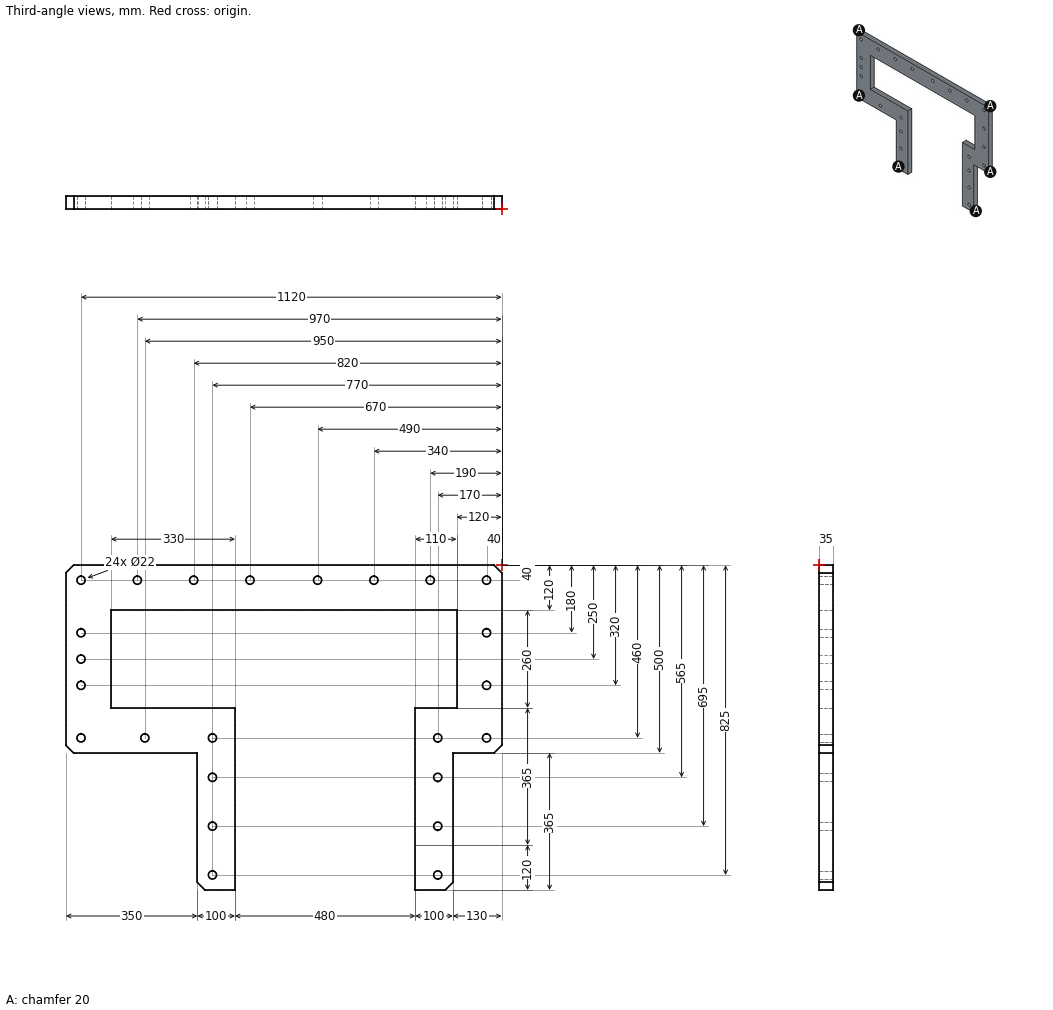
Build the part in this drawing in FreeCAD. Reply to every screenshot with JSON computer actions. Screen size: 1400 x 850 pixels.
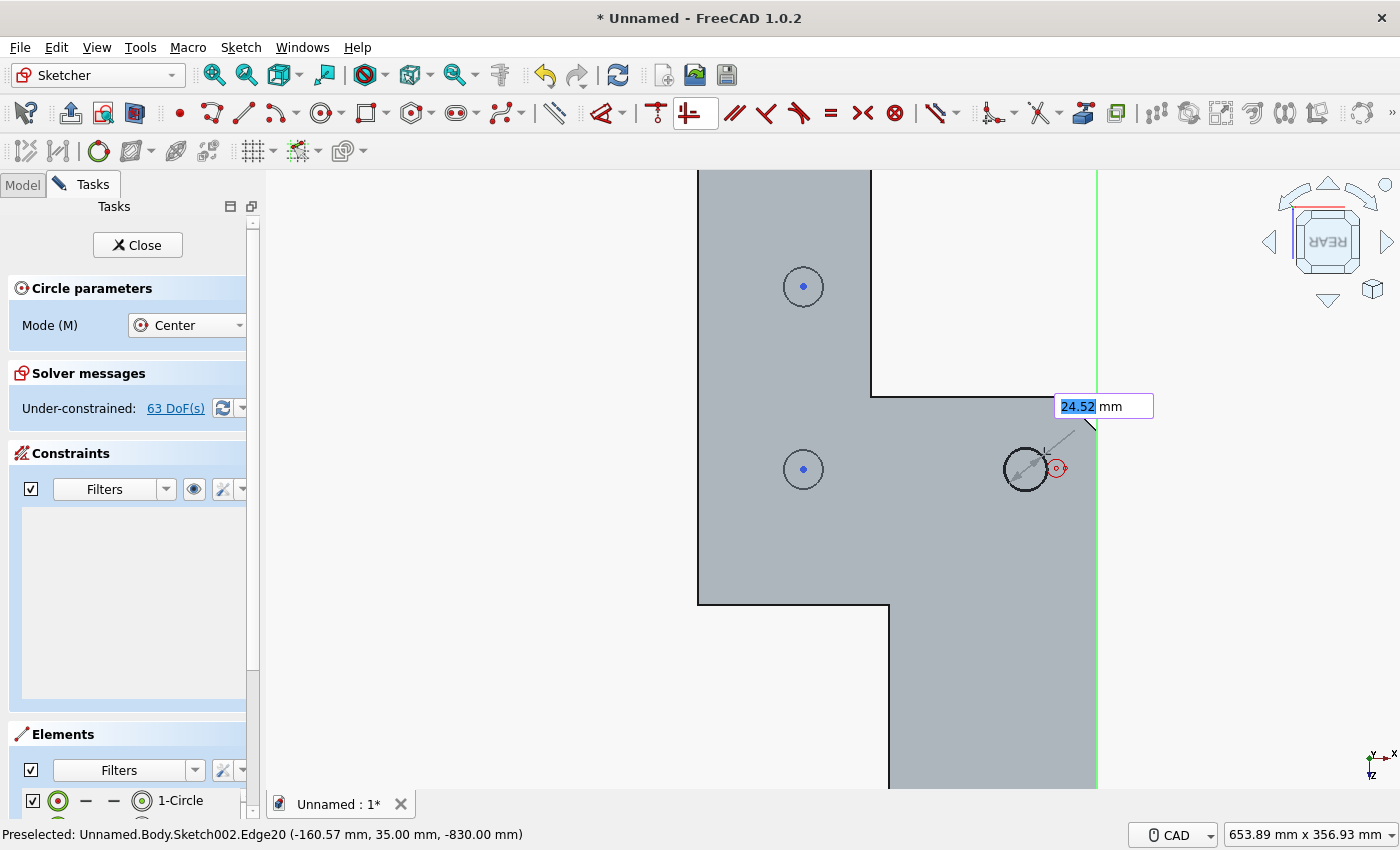
{"action": "left_click", "coordinate": [1041, 453]}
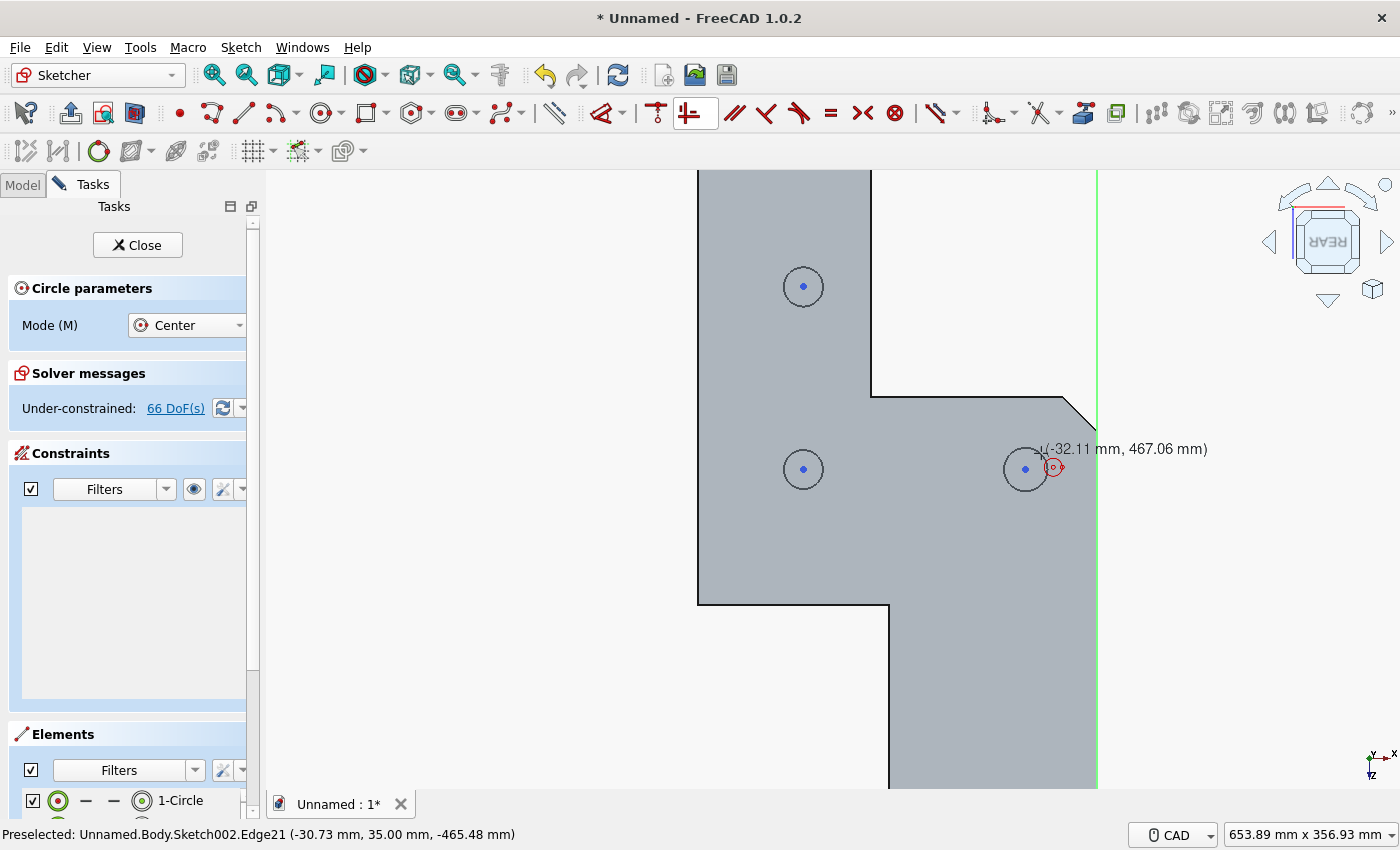
{"action": "scroll", "coordinate": [1044, 454], "scroll_direction": "down", "scroll_amount": 6}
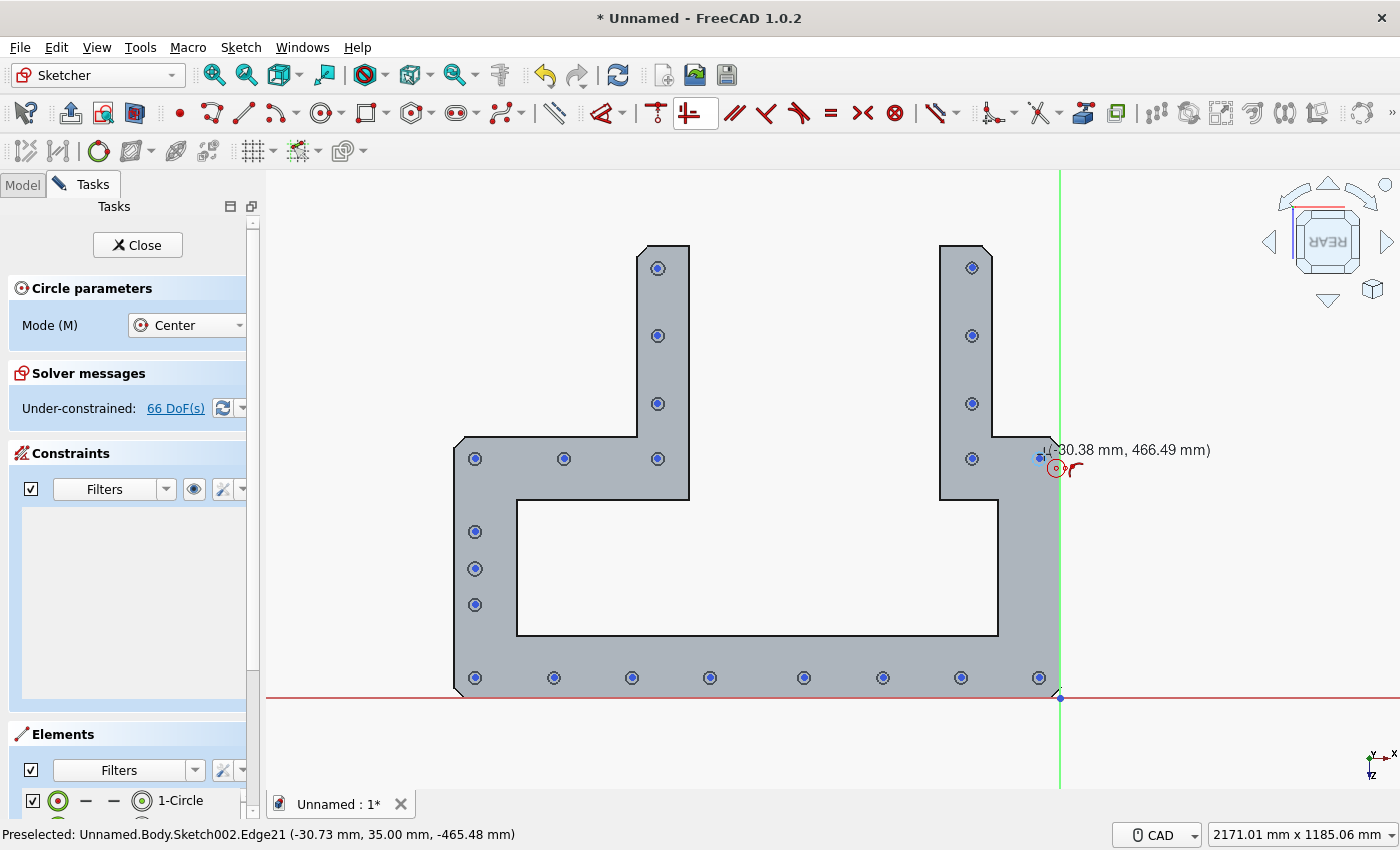
{"action": "left_click", "coordinate": [1039, 531]}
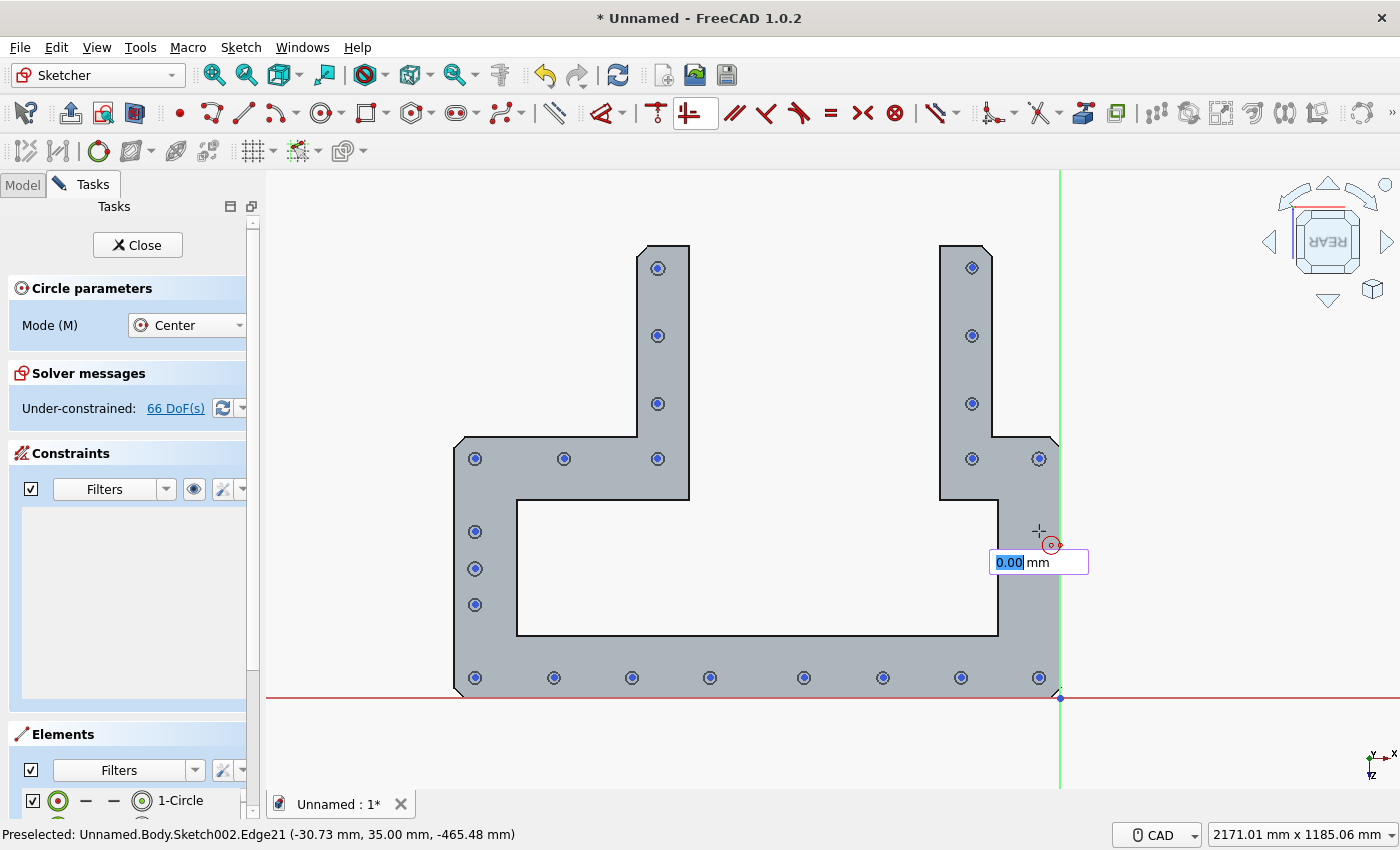
{"action": "scroll", "coordinate": [1044, 527], "scroll_direction": "up", "scroll_amount": 6}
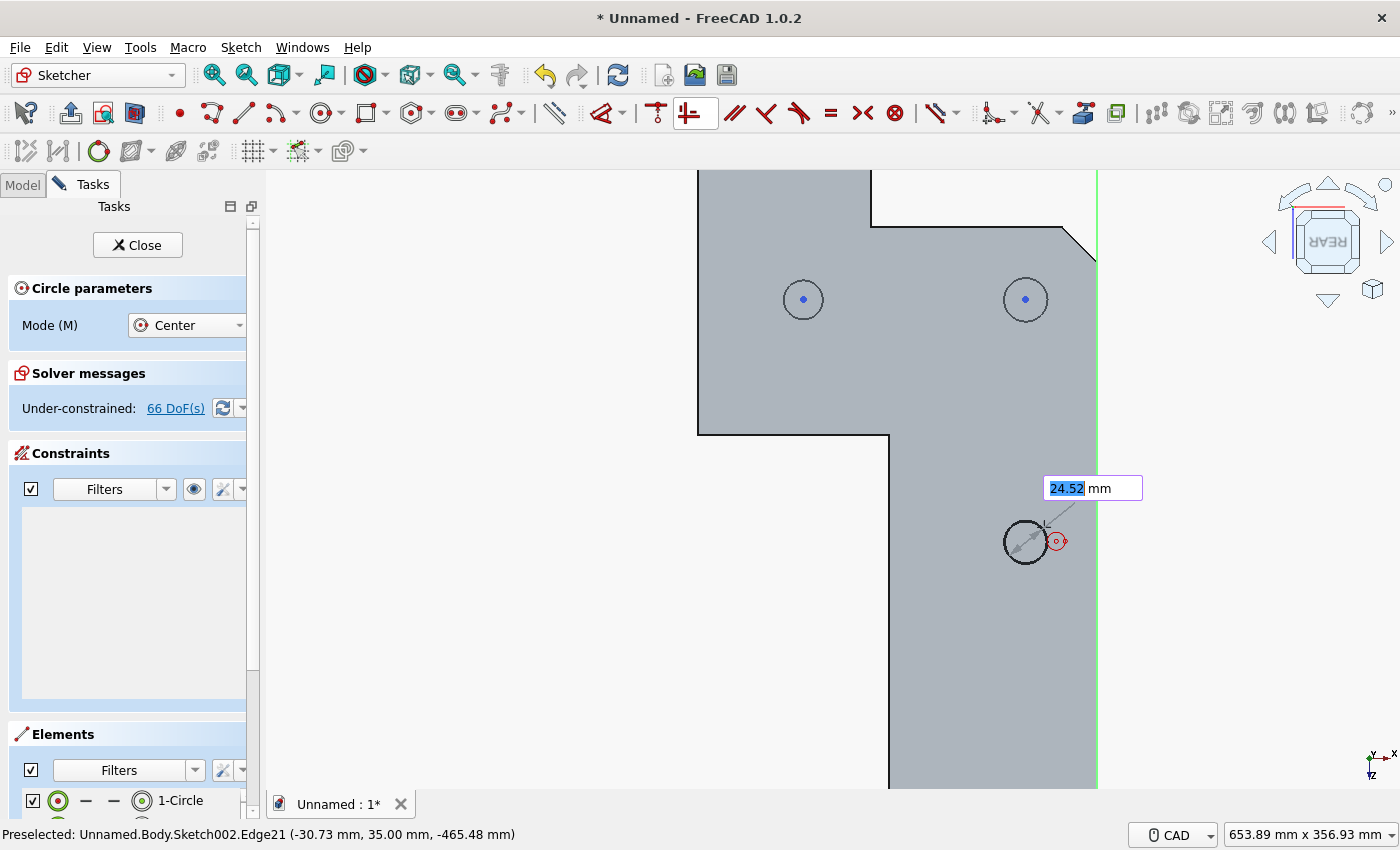
{"action": "left_click", "coordinate": [1041, 526]}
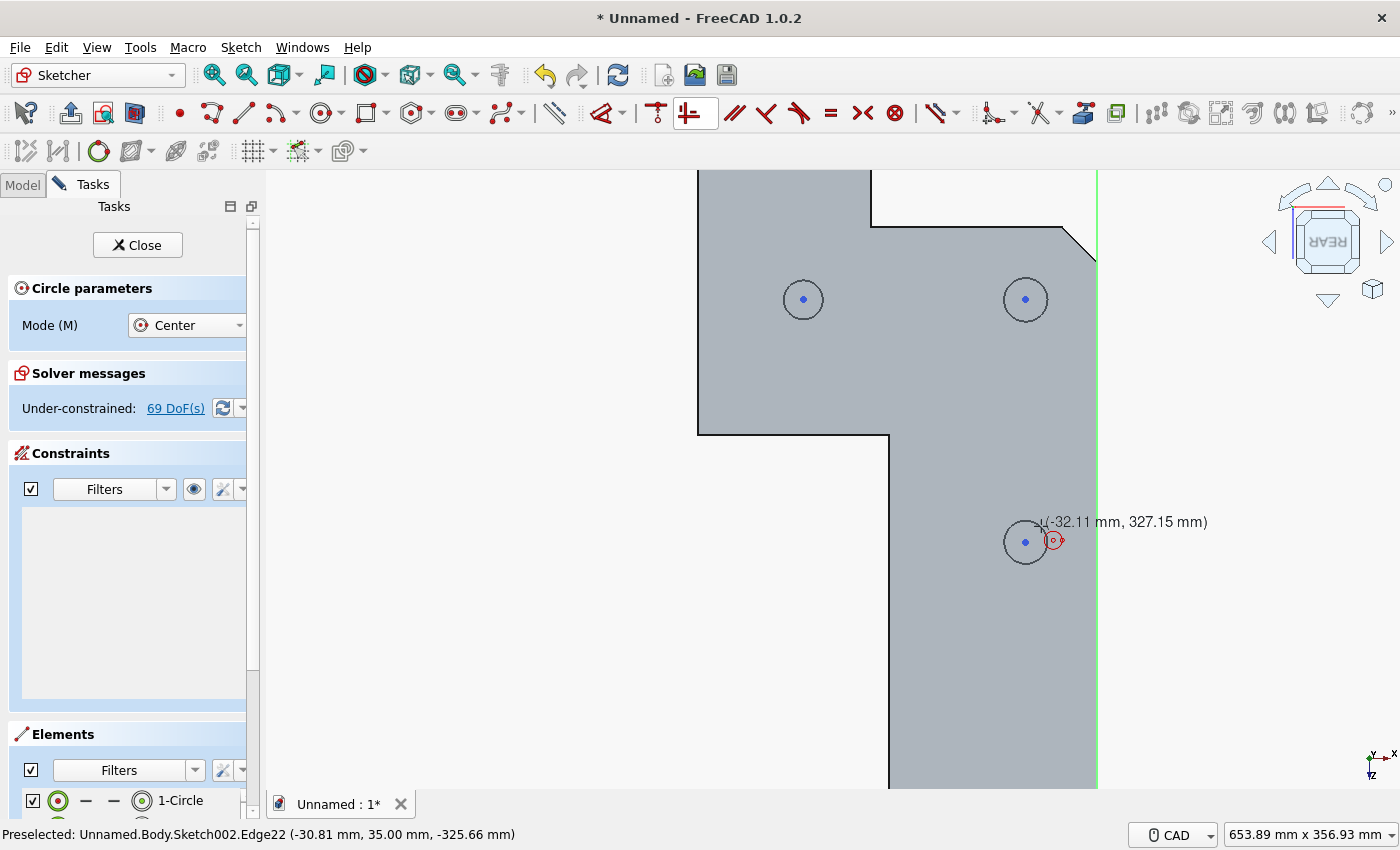
{"action": "scroll", "coordinate": [1044, 527], "scroll_direction": "down", "scroll_amount": 6}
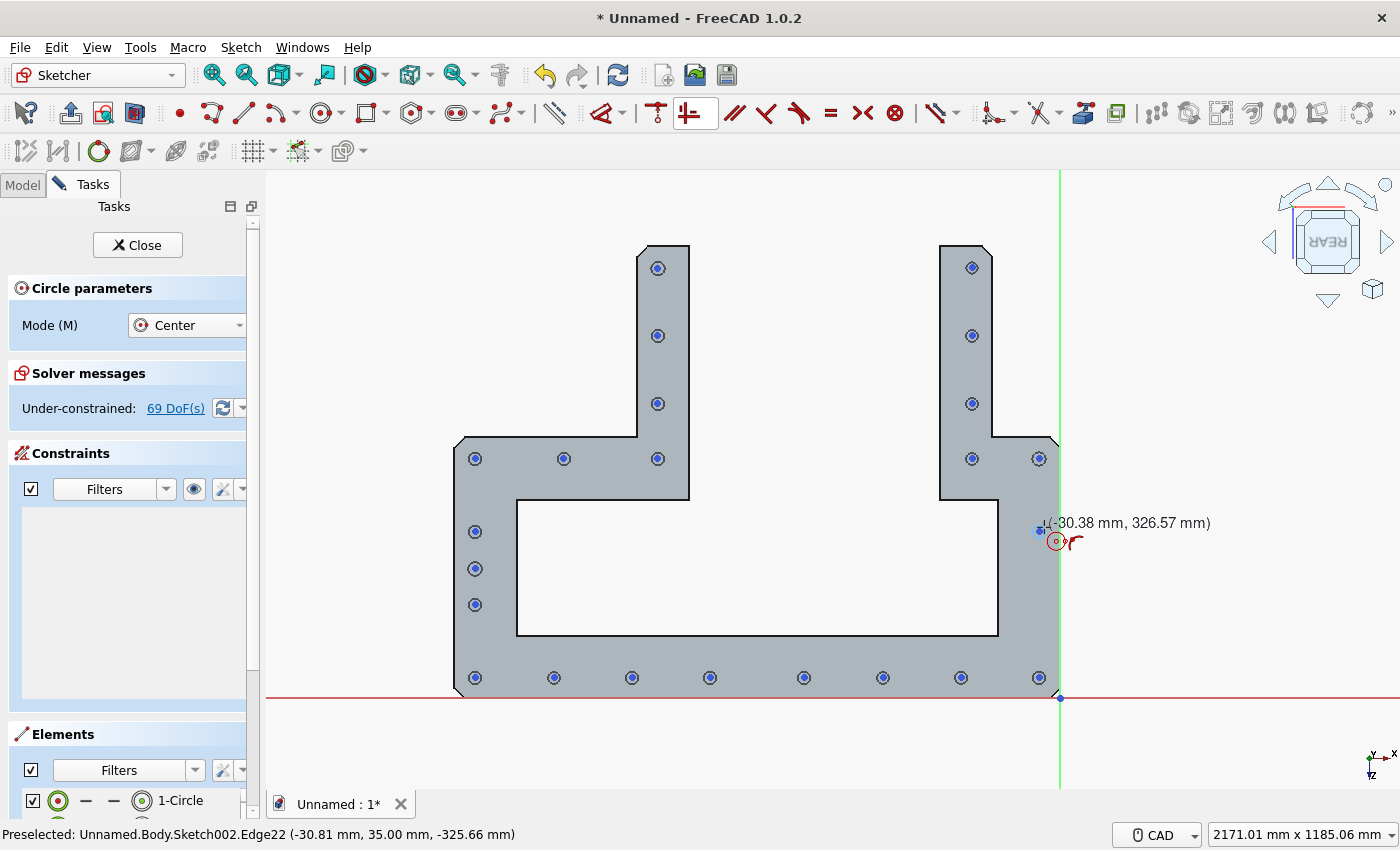
{"action": "scroll", "coordinate": [1039, 604], "scroll_direction": "up", "scroll_amount": 7}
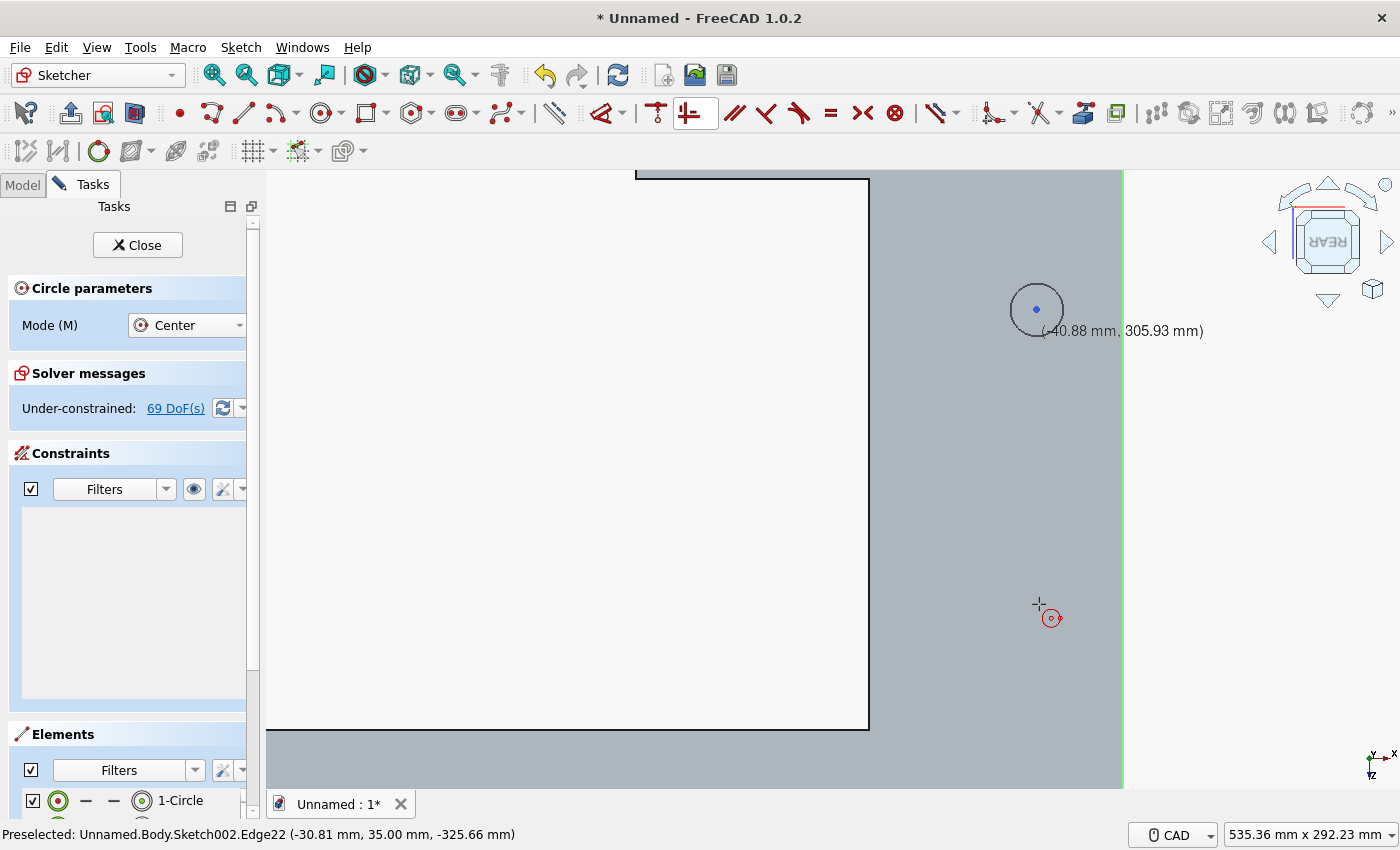
{"action": "scroll", "coordinate": [1039, 604], "scroll_direction": "down", "scroll_amount": 7}